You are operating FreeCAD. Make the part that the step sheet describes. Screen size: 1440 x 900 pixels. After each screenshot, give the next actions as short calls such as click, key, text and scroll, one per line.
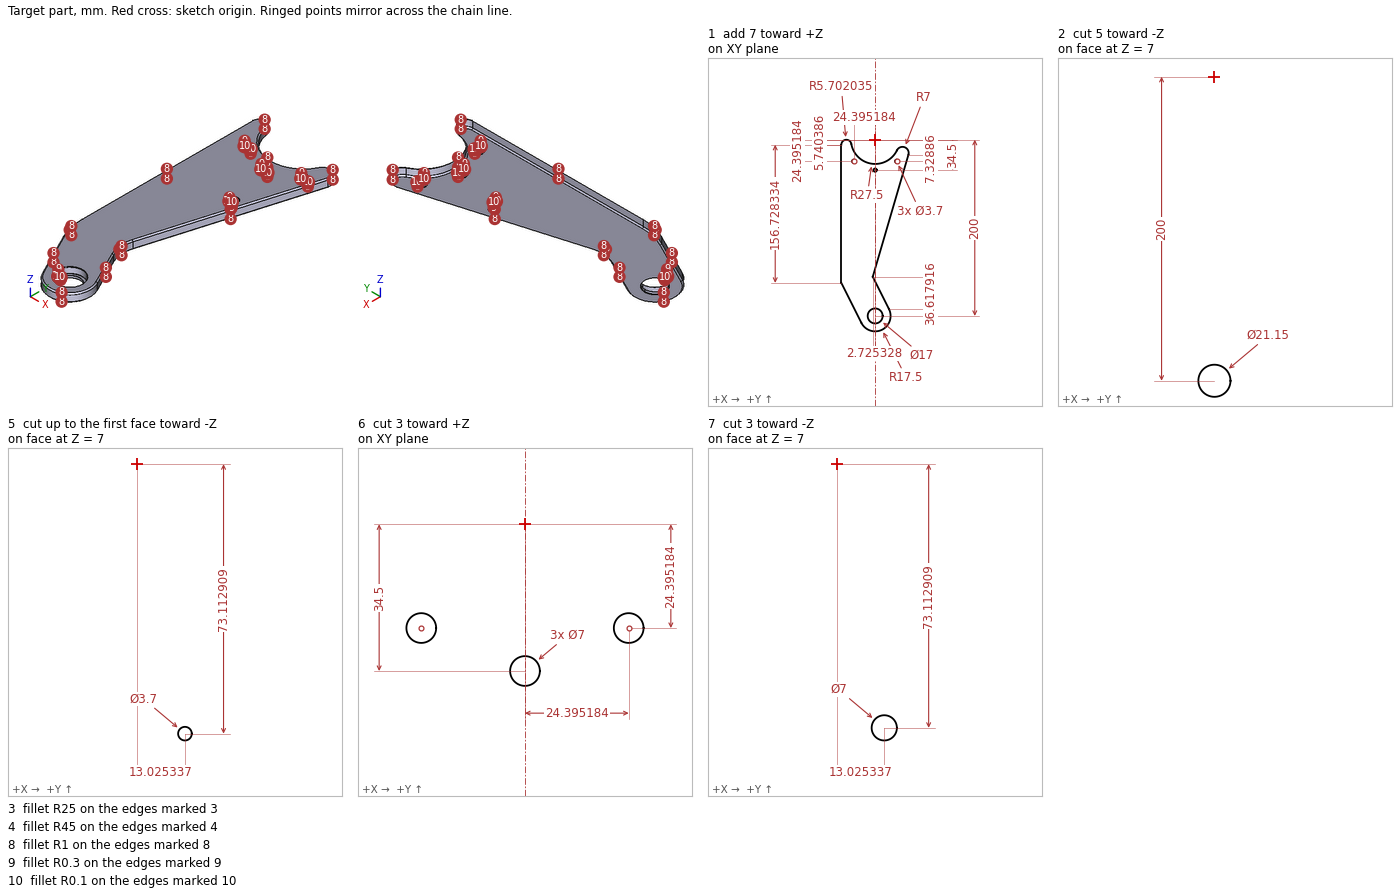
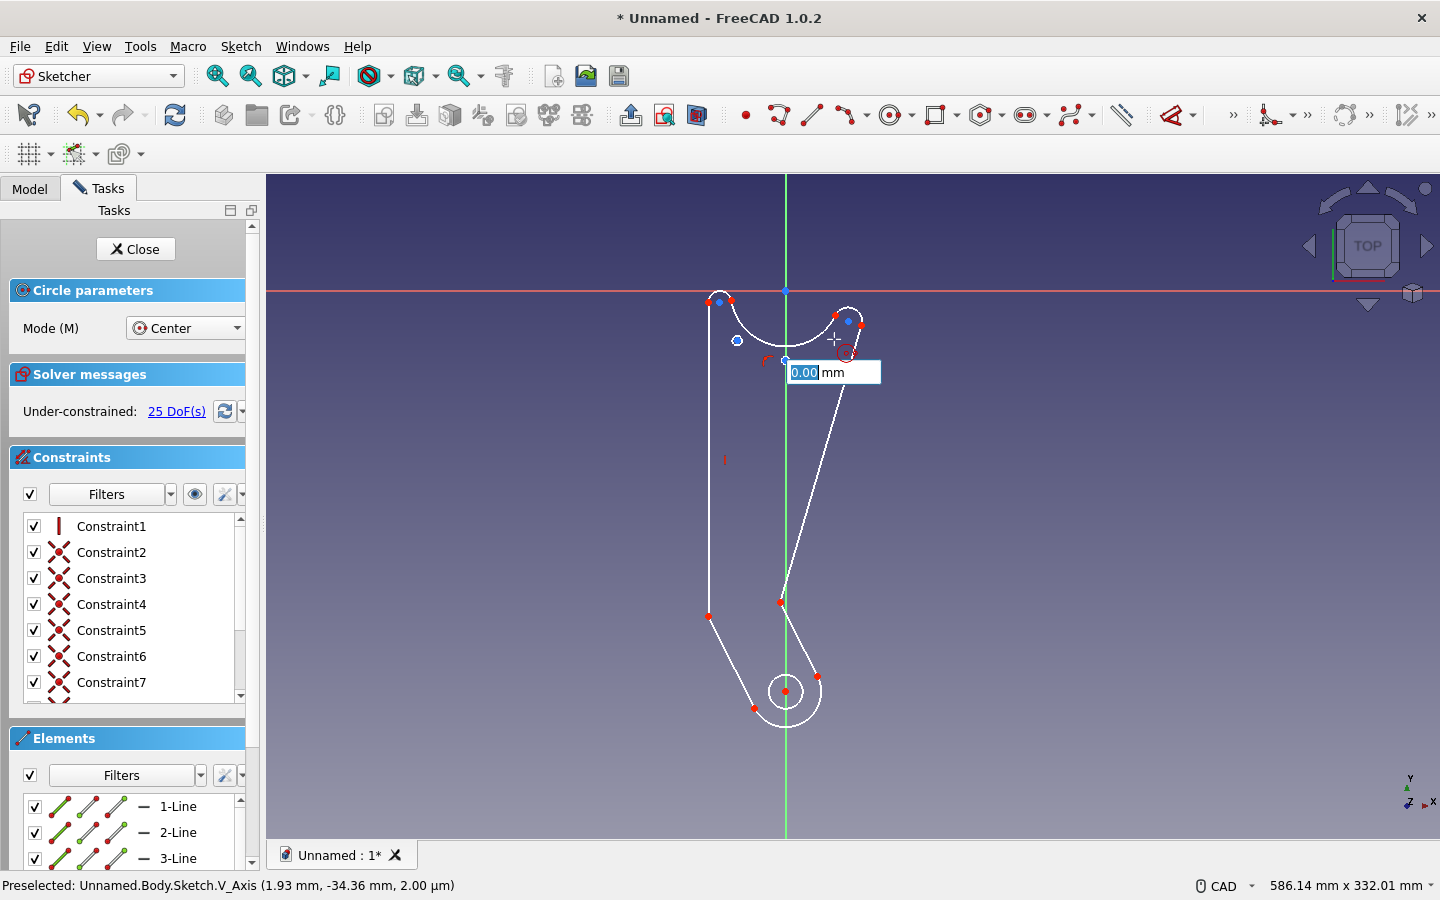
scroll(837, 337, up, 8)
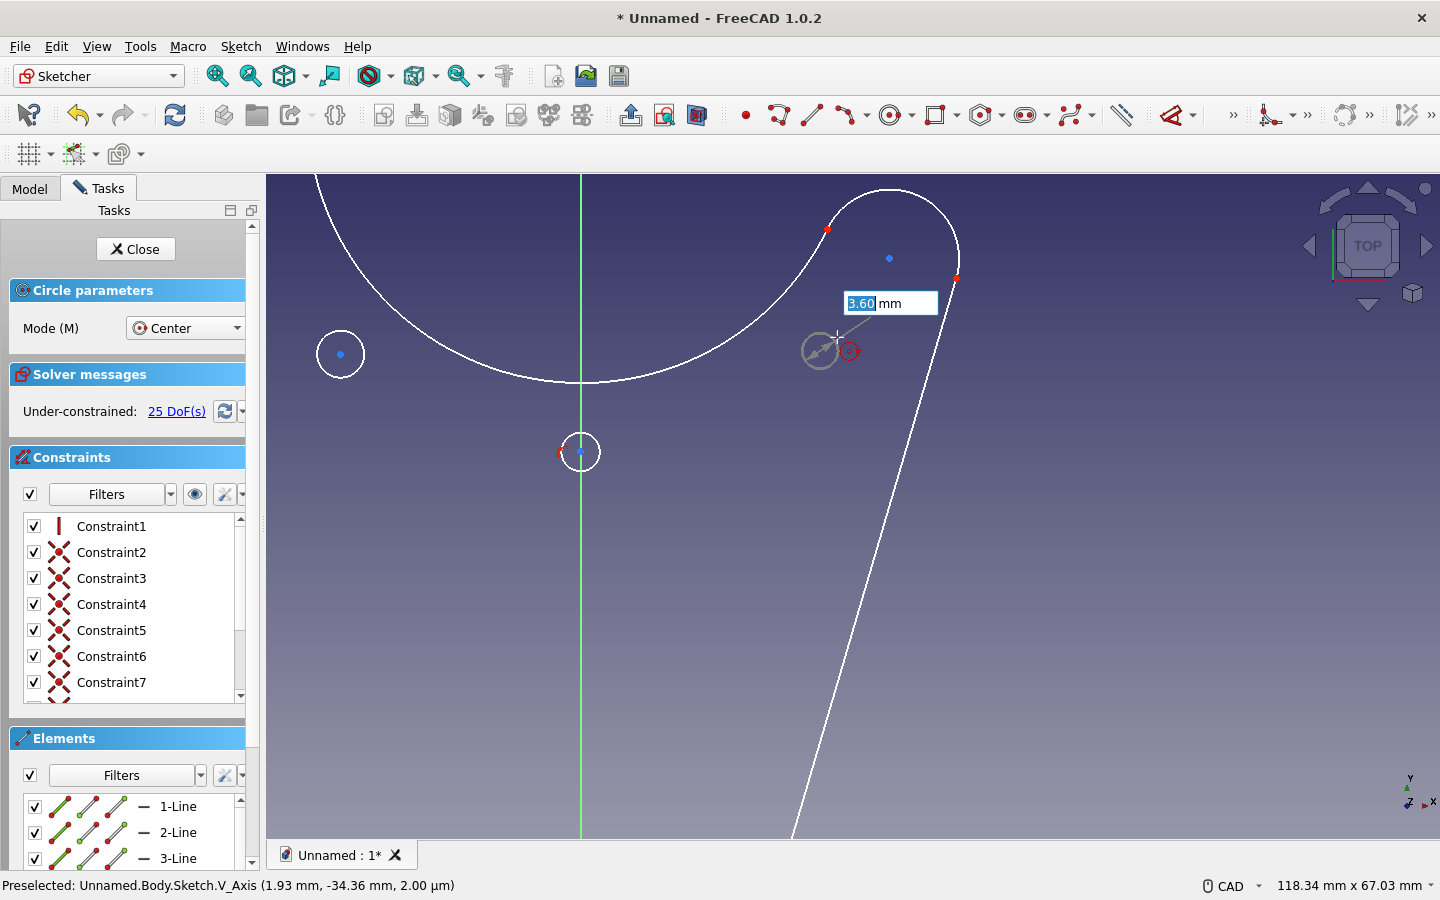
click(836, 335)
key(Escape)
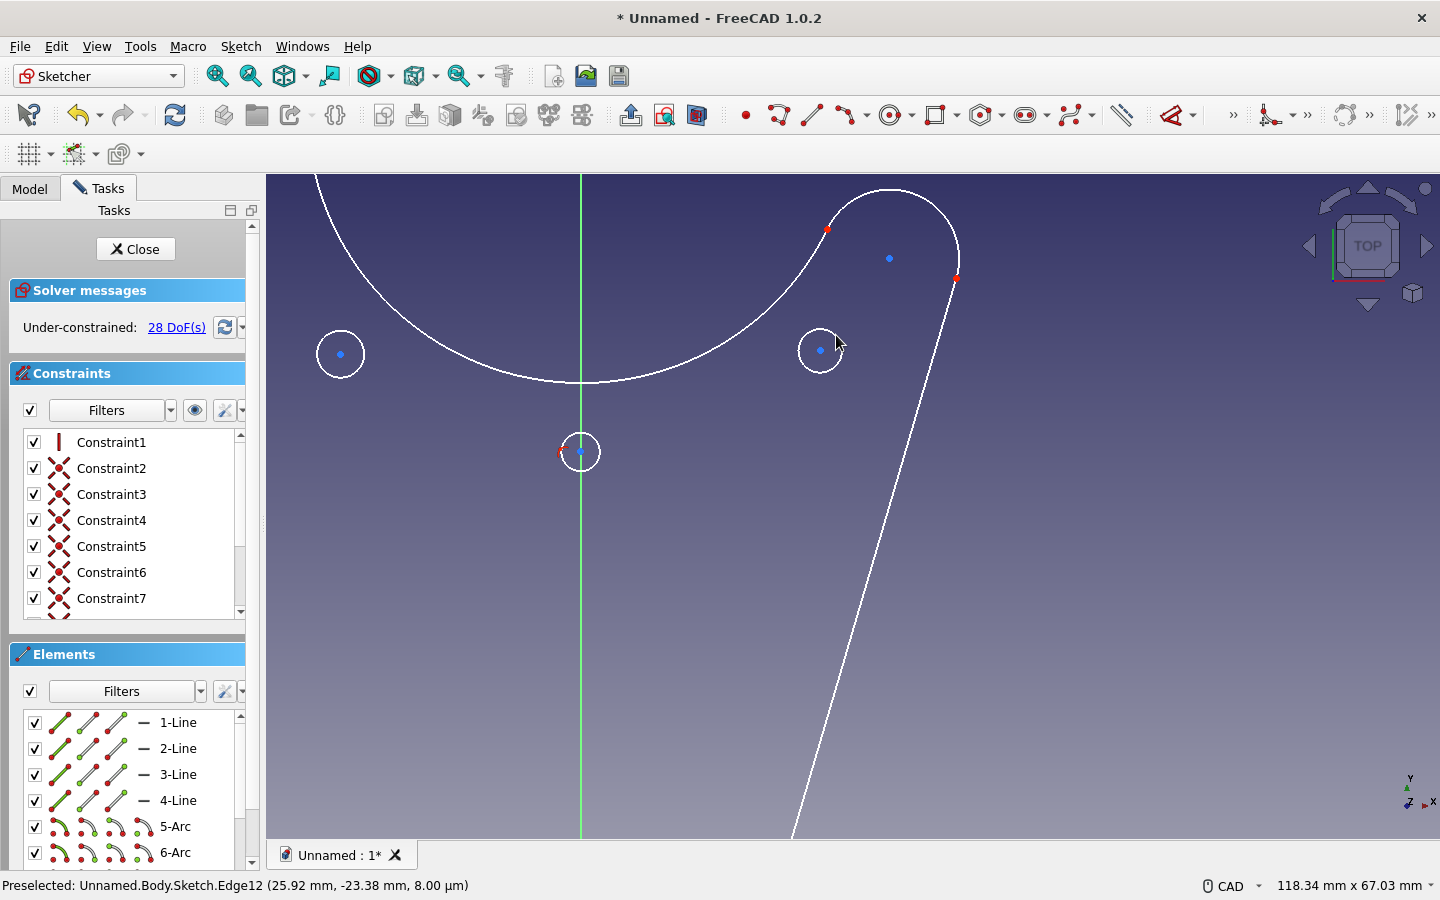
scroll(837, 337, down, 8)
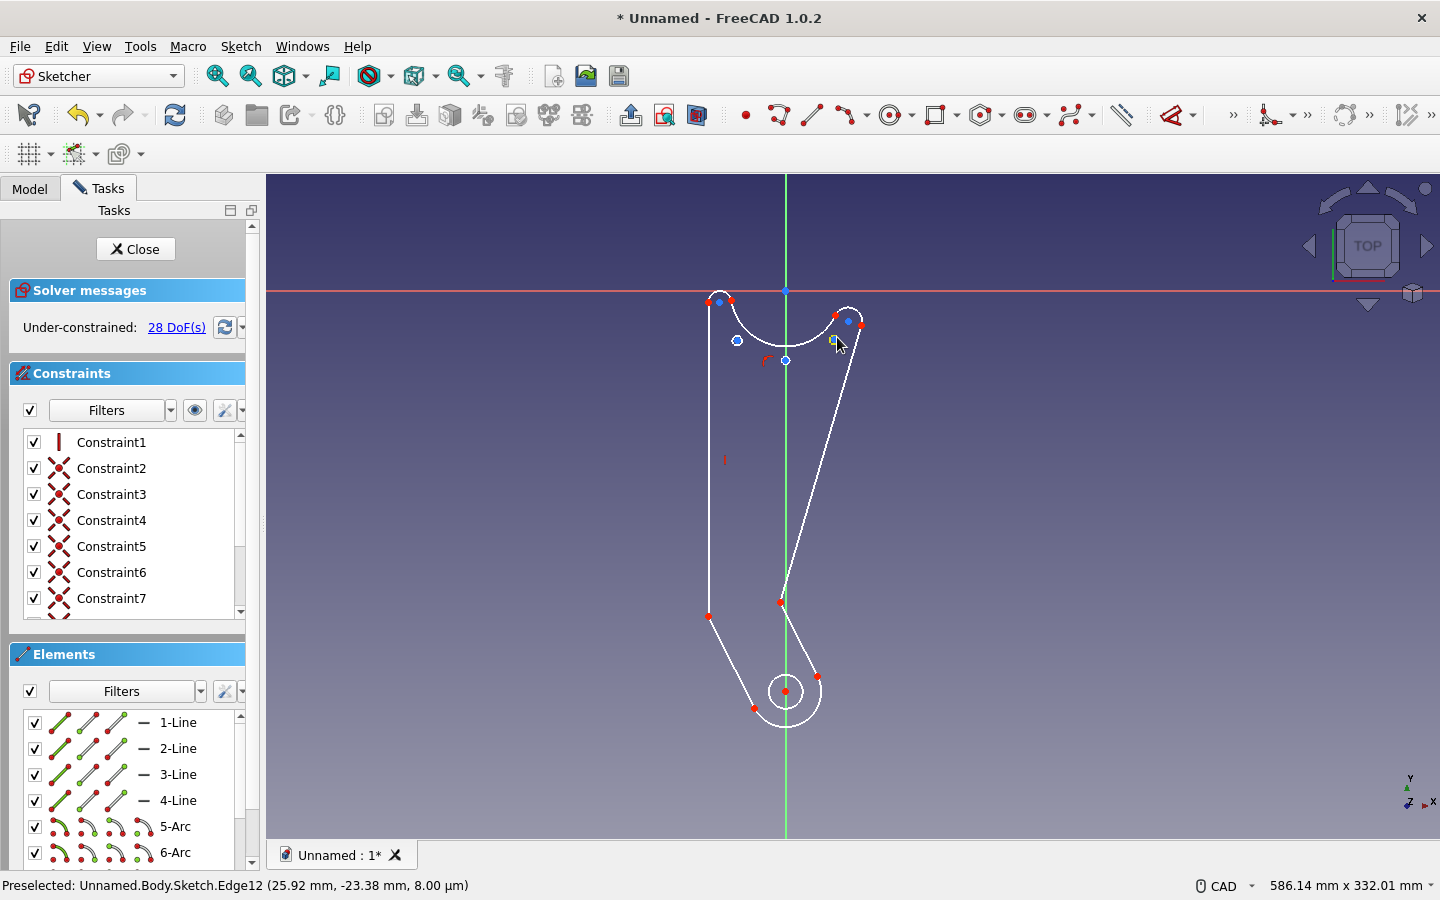
click(709, 397)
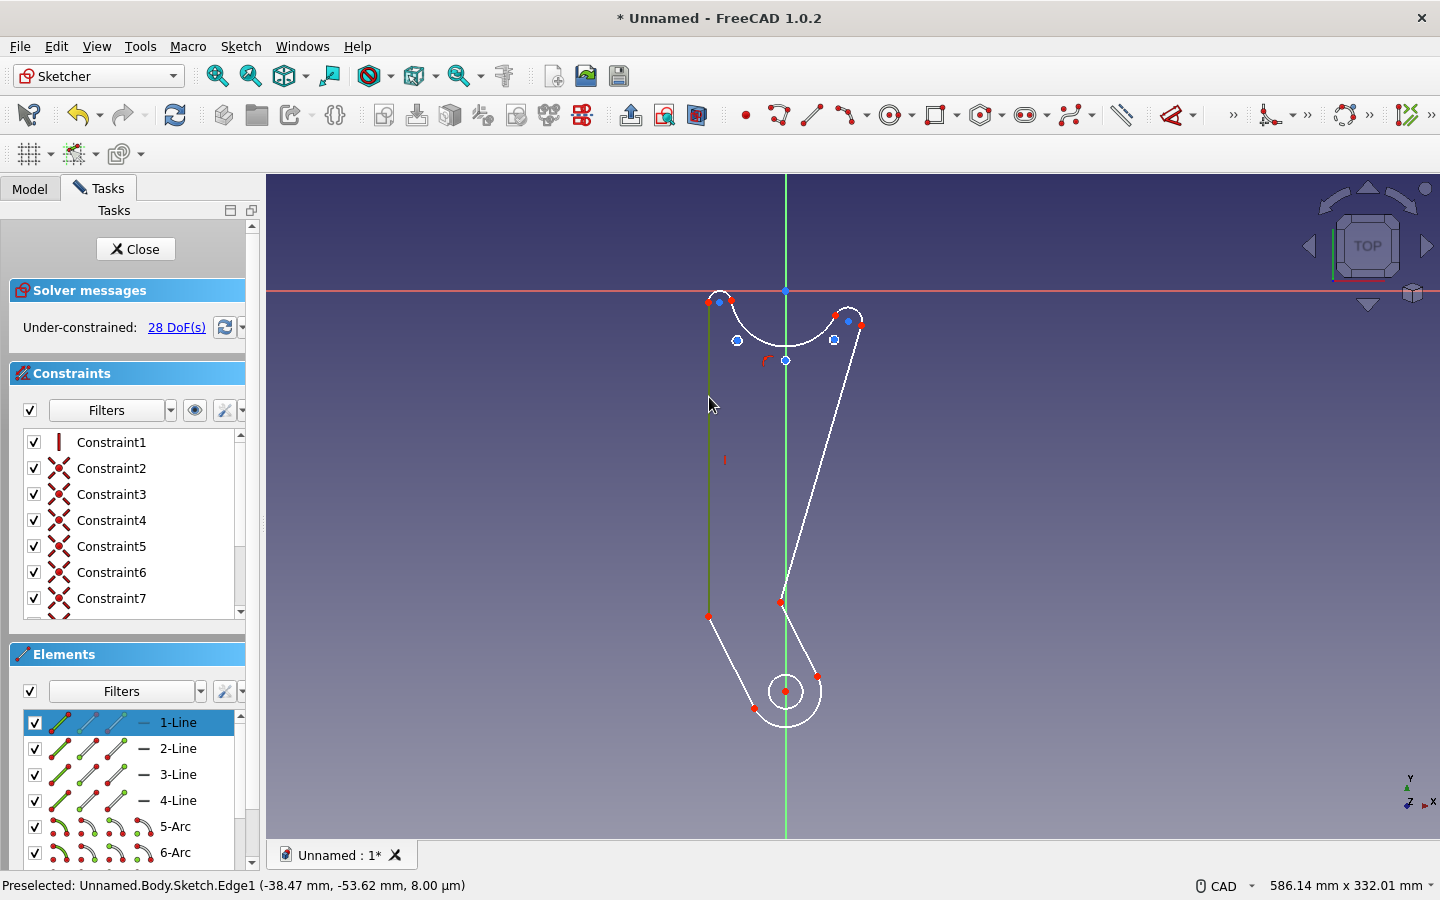
scroll(726, 293, up, 2)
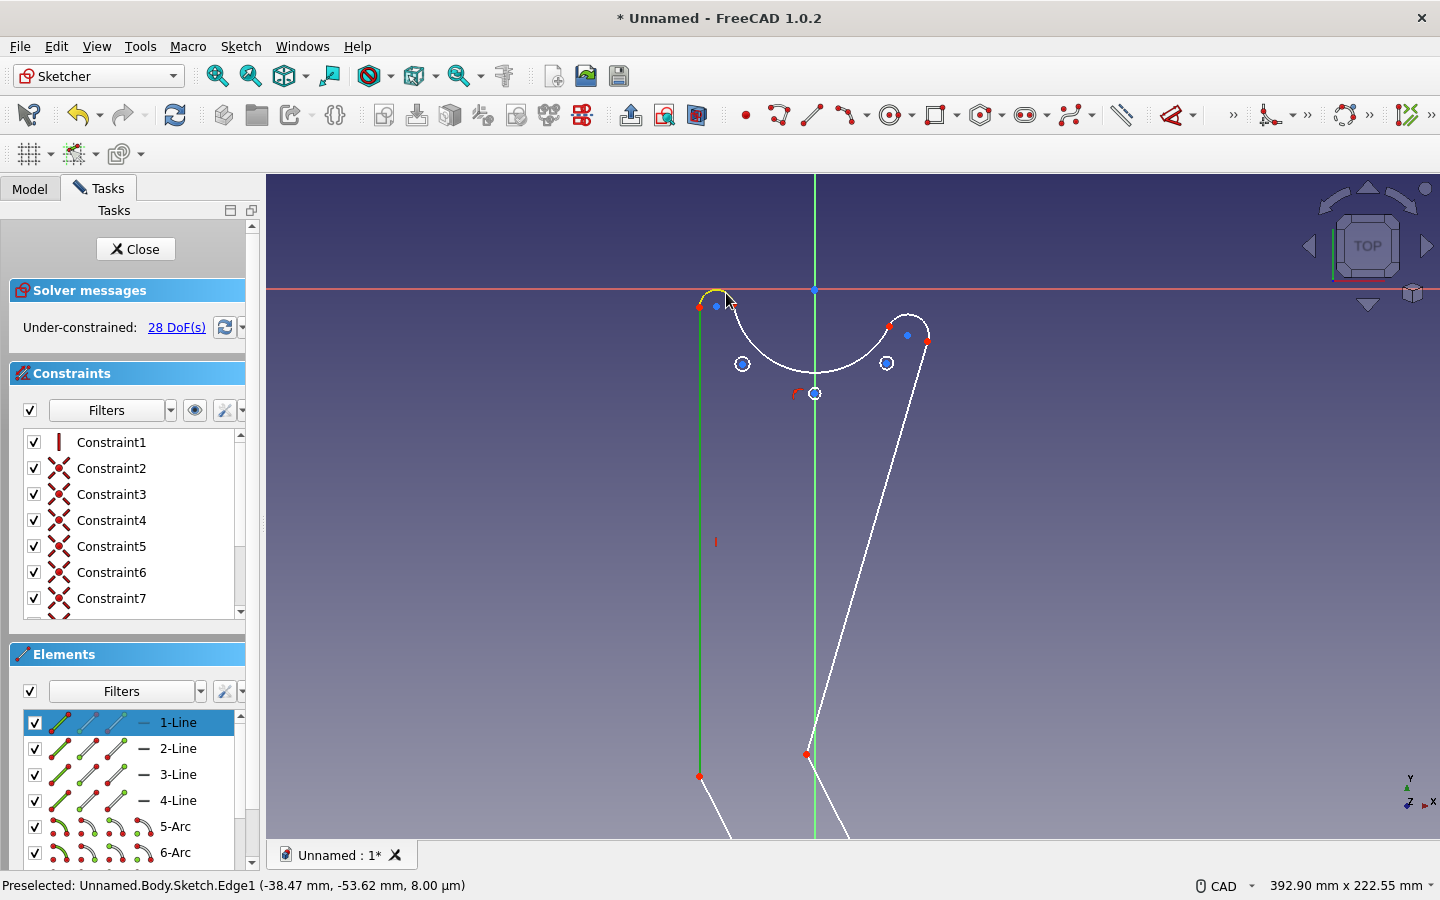
click(725, 292)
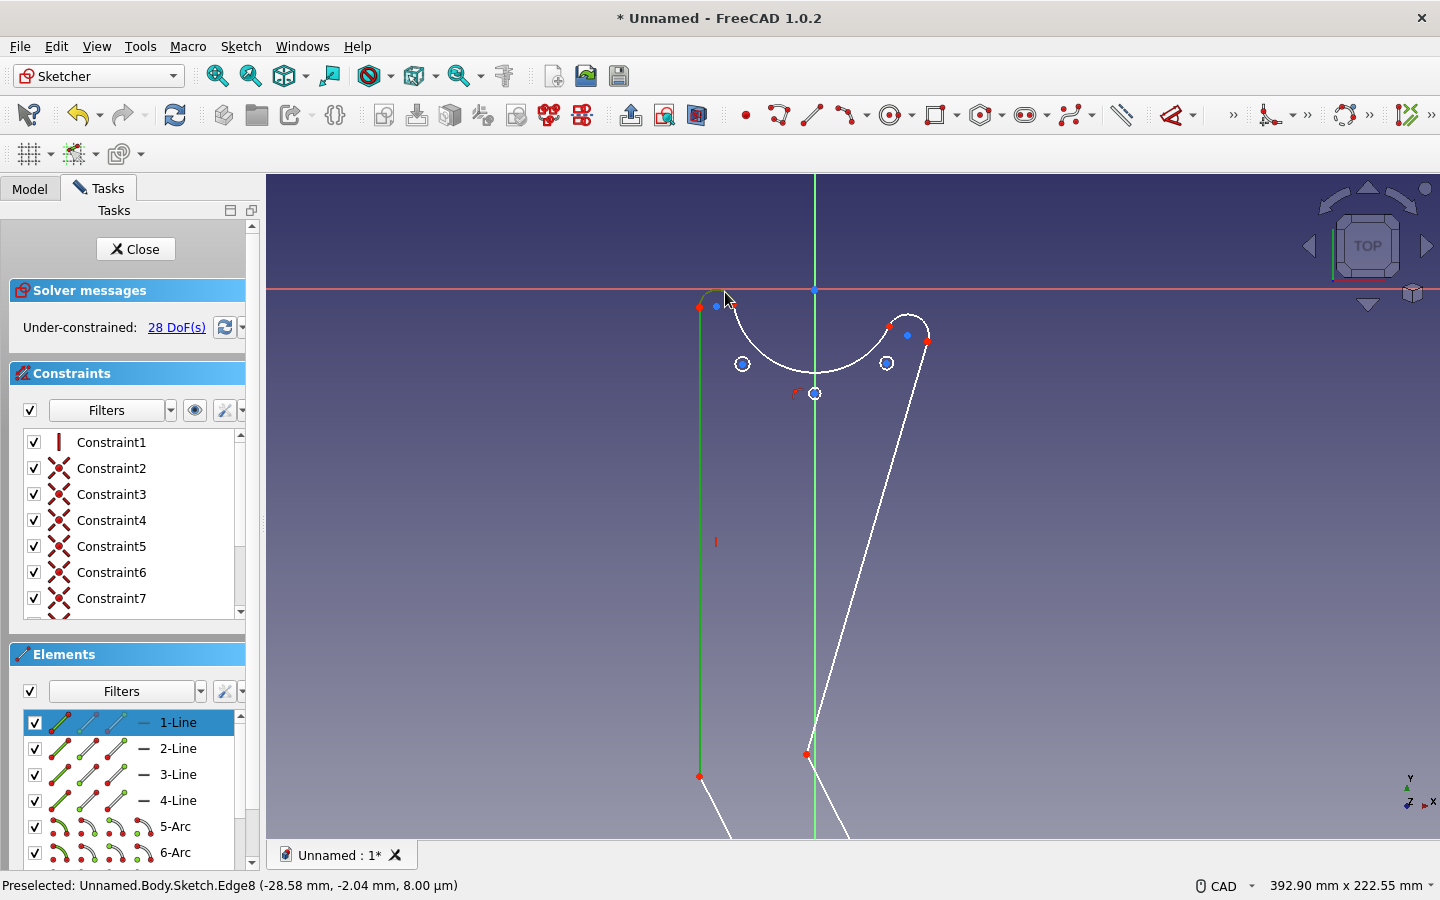
key(t)